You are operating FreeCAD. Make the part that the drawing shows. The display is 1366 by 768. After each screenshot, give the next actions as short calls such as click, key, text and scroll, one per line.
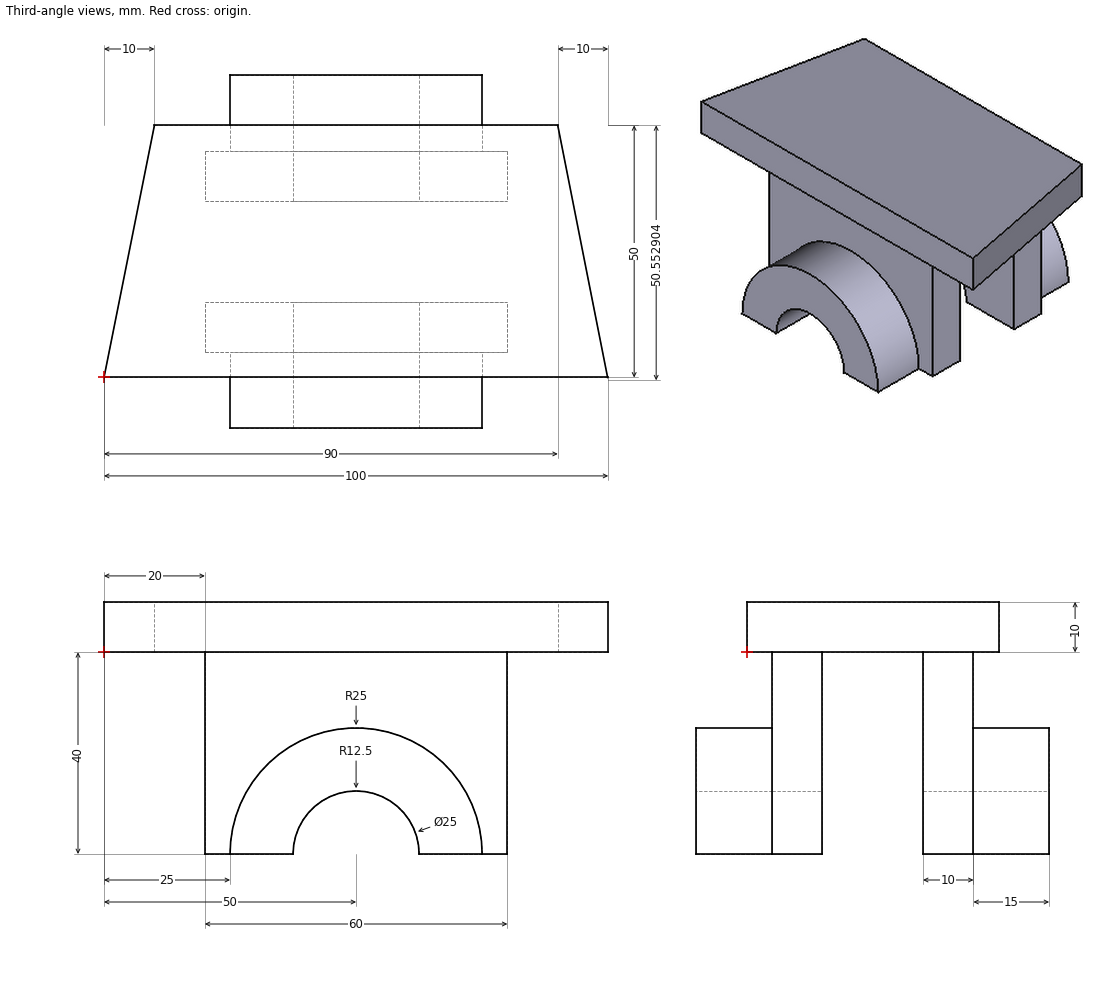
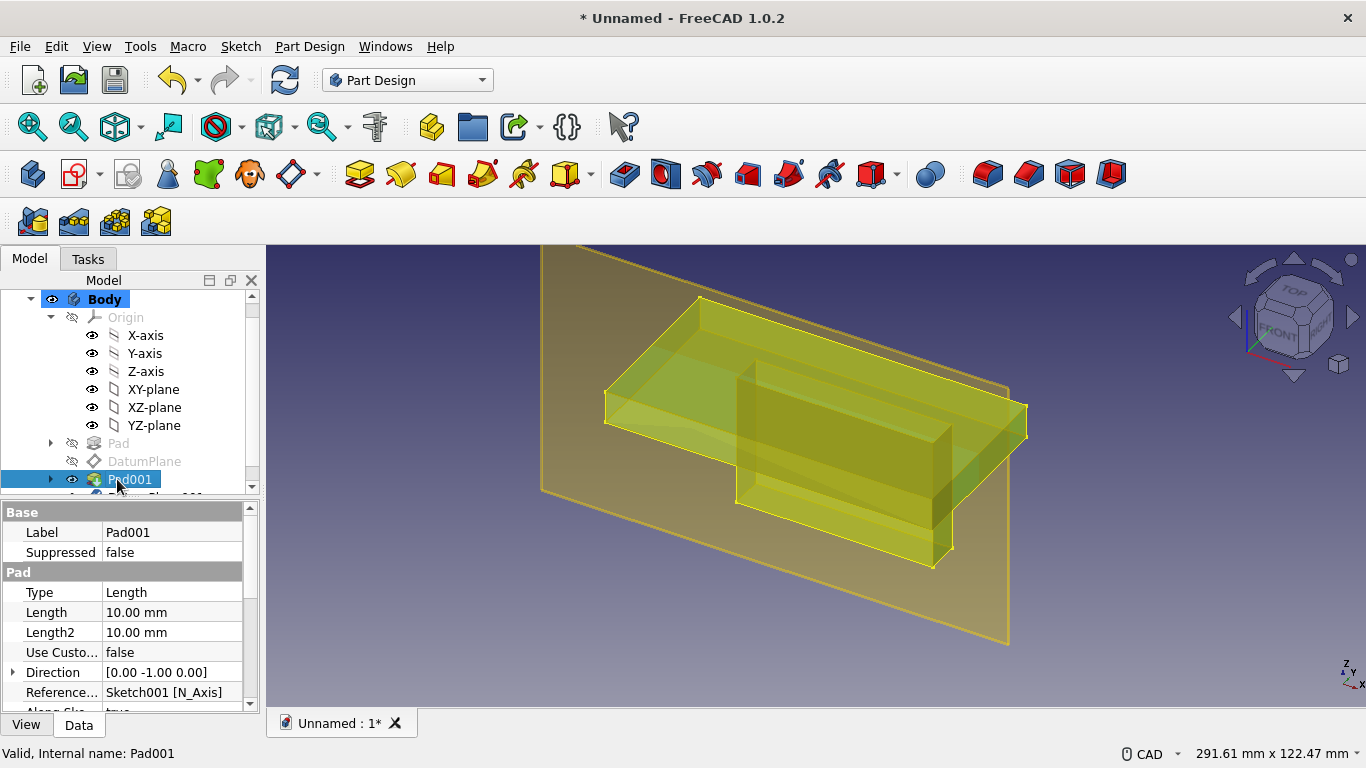
click(33, 222)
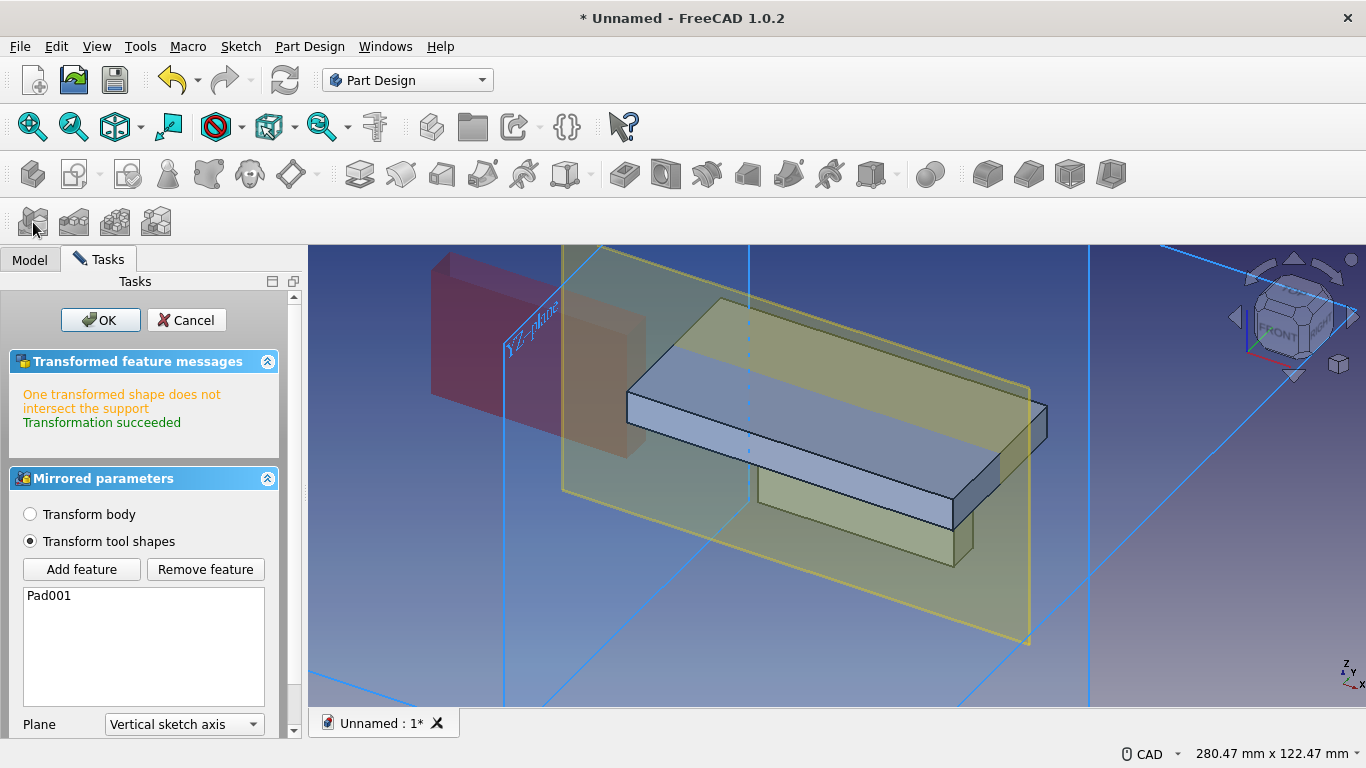
click(185, 724)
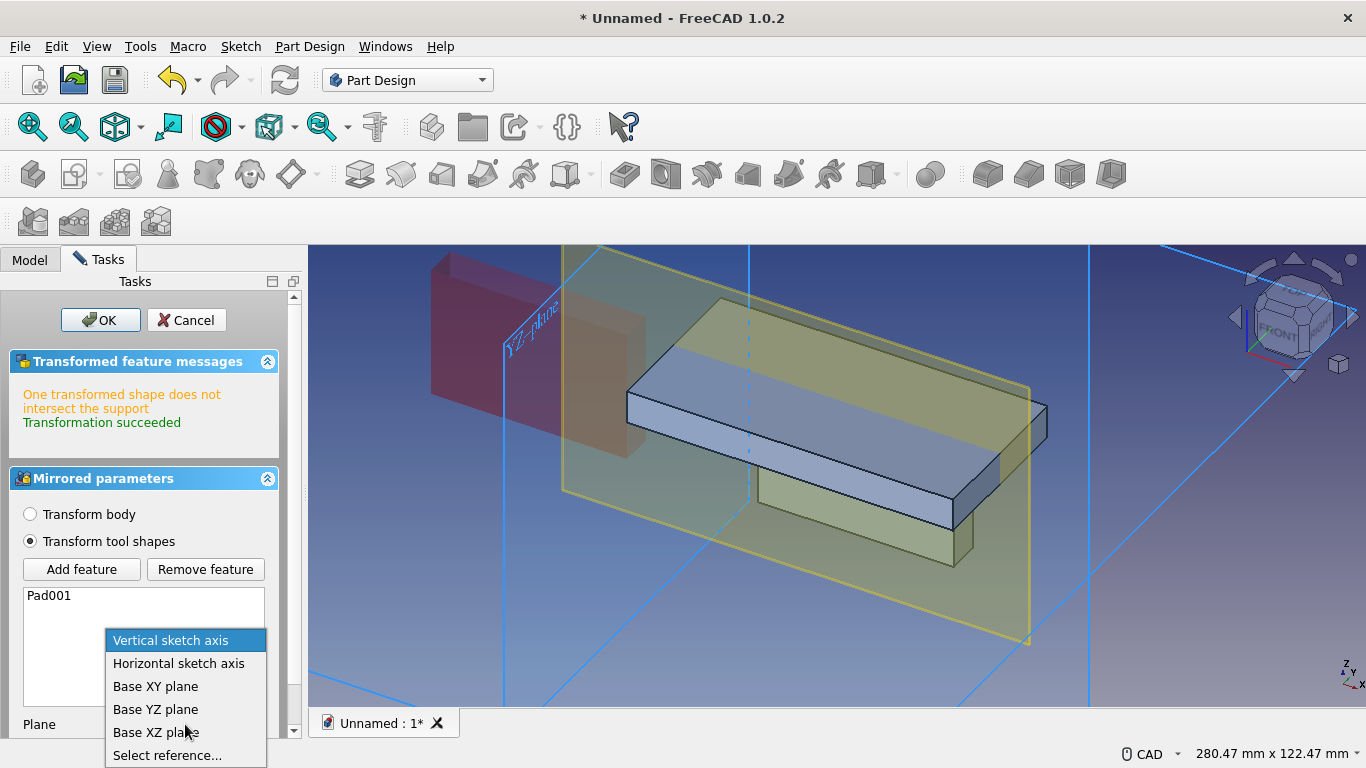
click(184, 756)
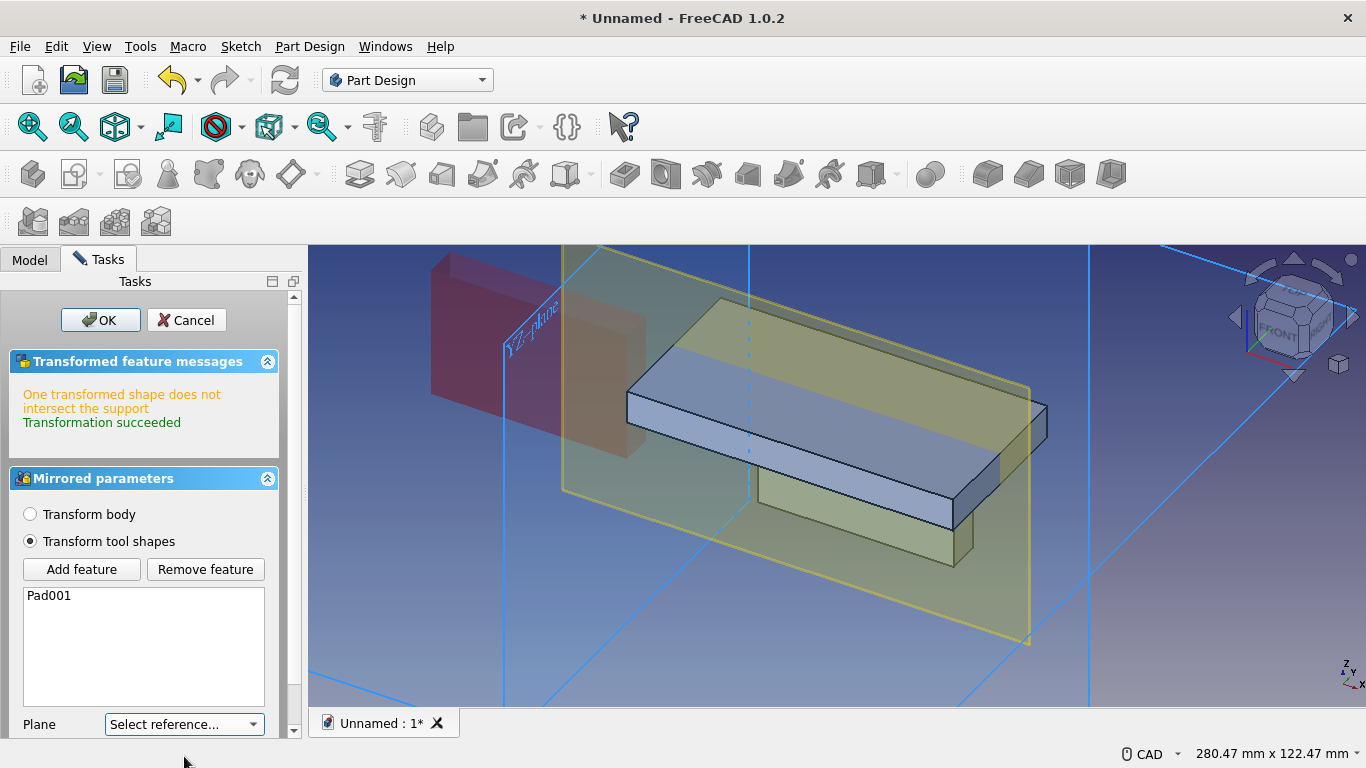
click(30, 259)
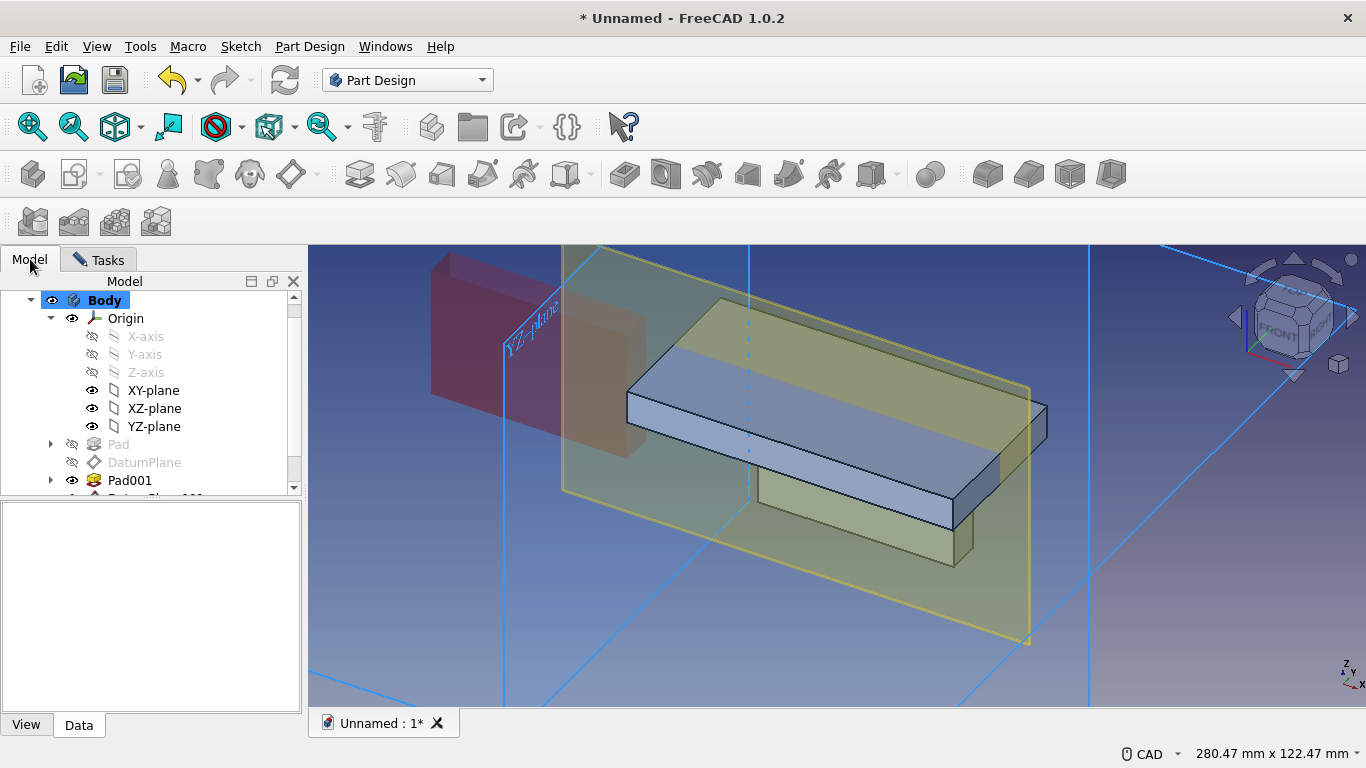
scroll(121, 386, down, 3)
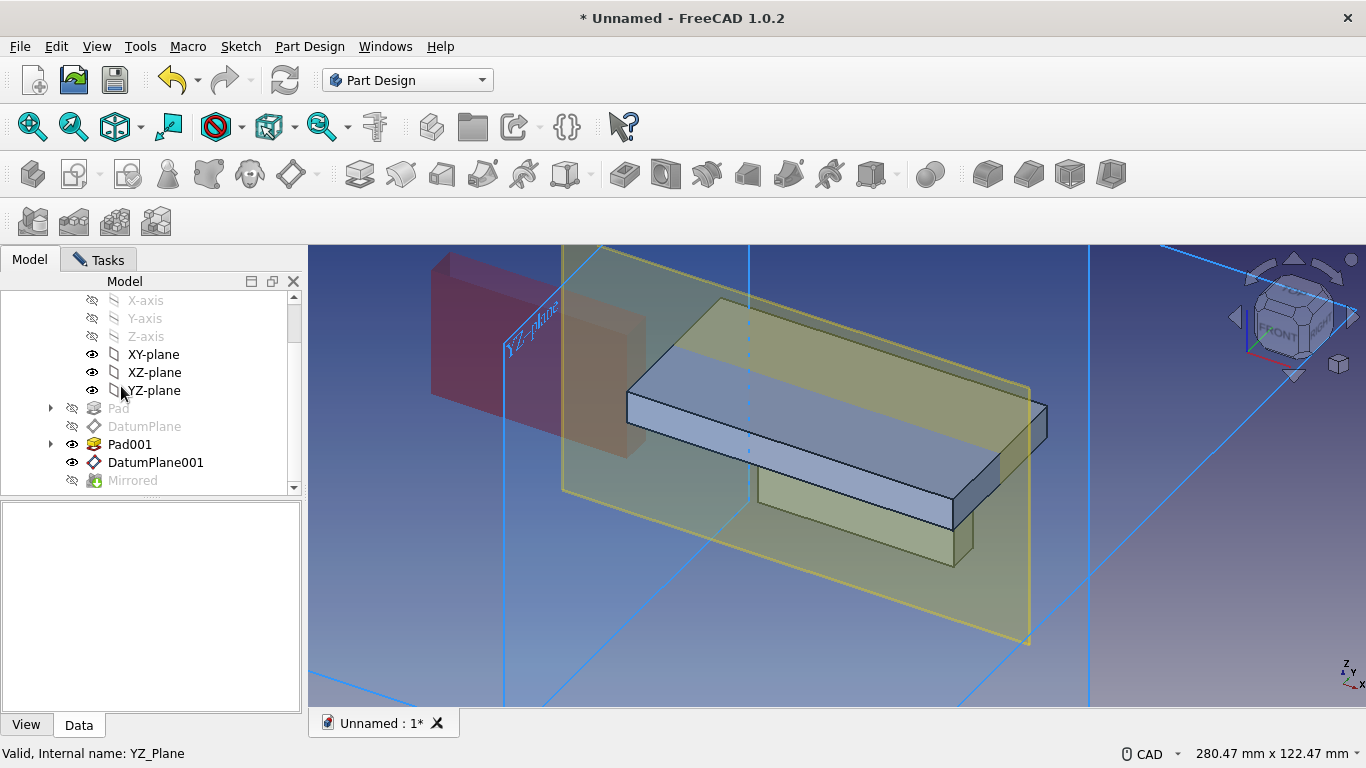
click(117, 462)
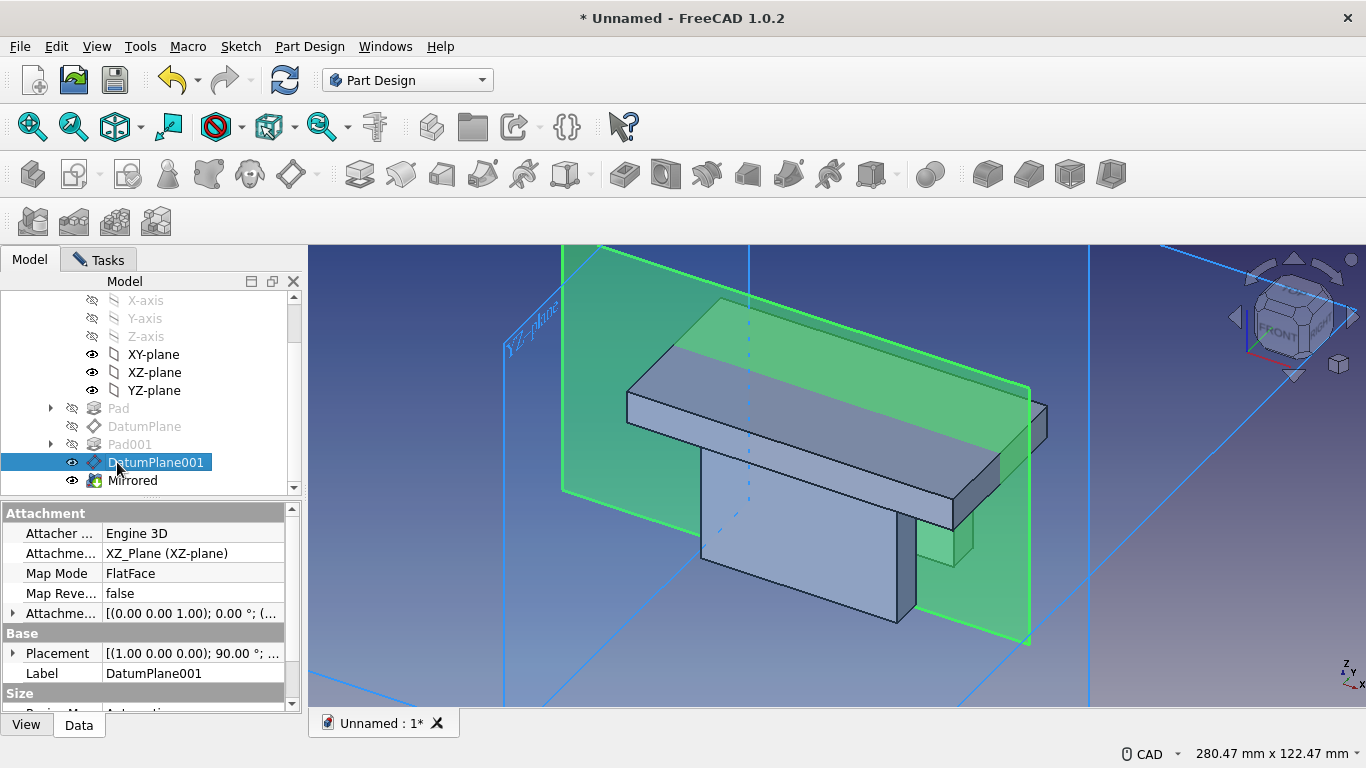
click(98, 259)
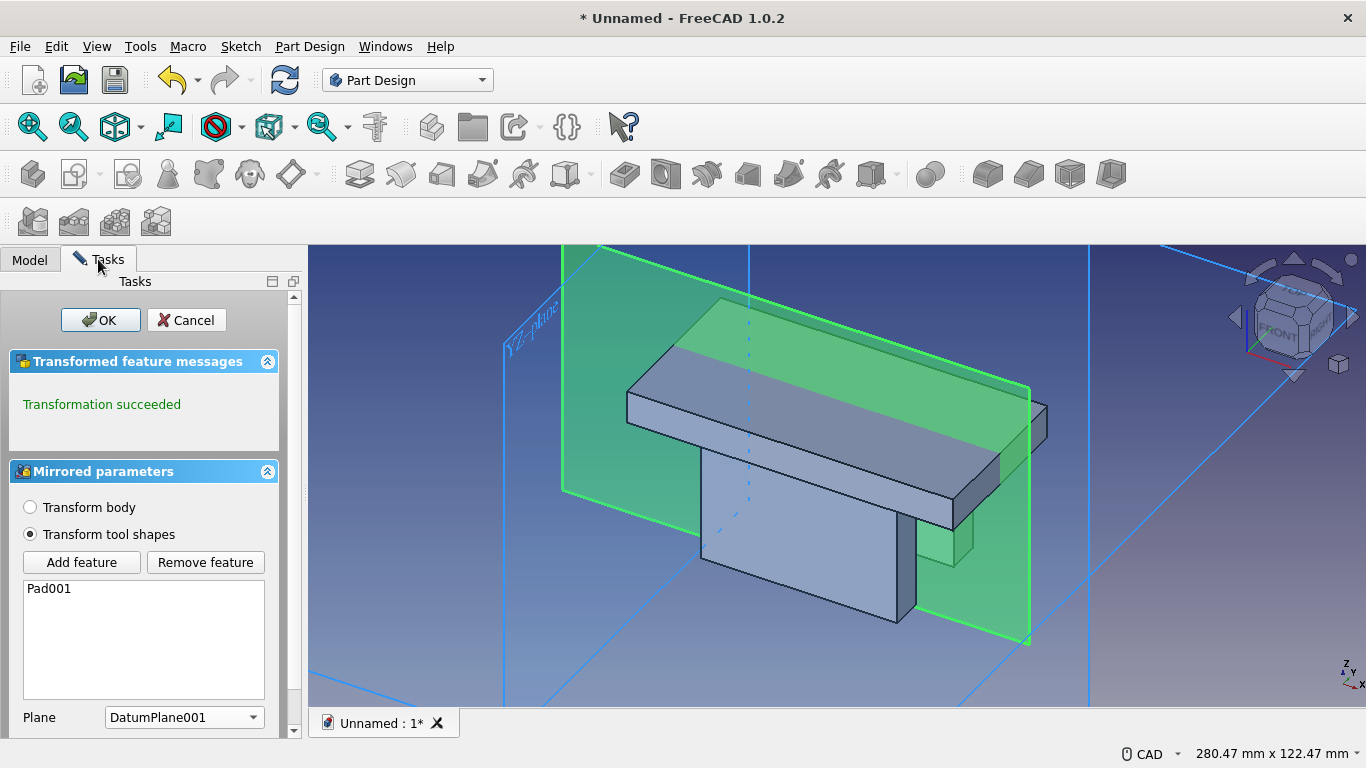
click(101, 320)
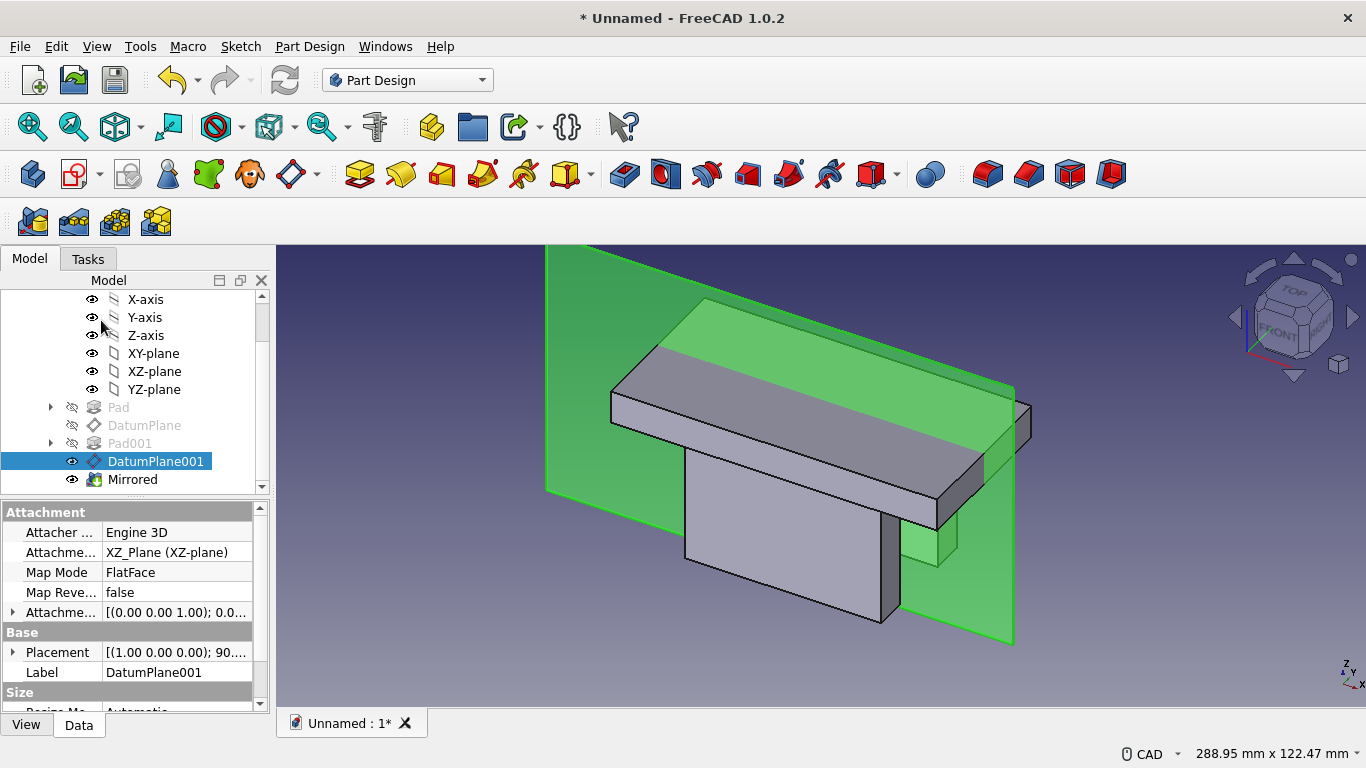
click(117, 461)
key(space)